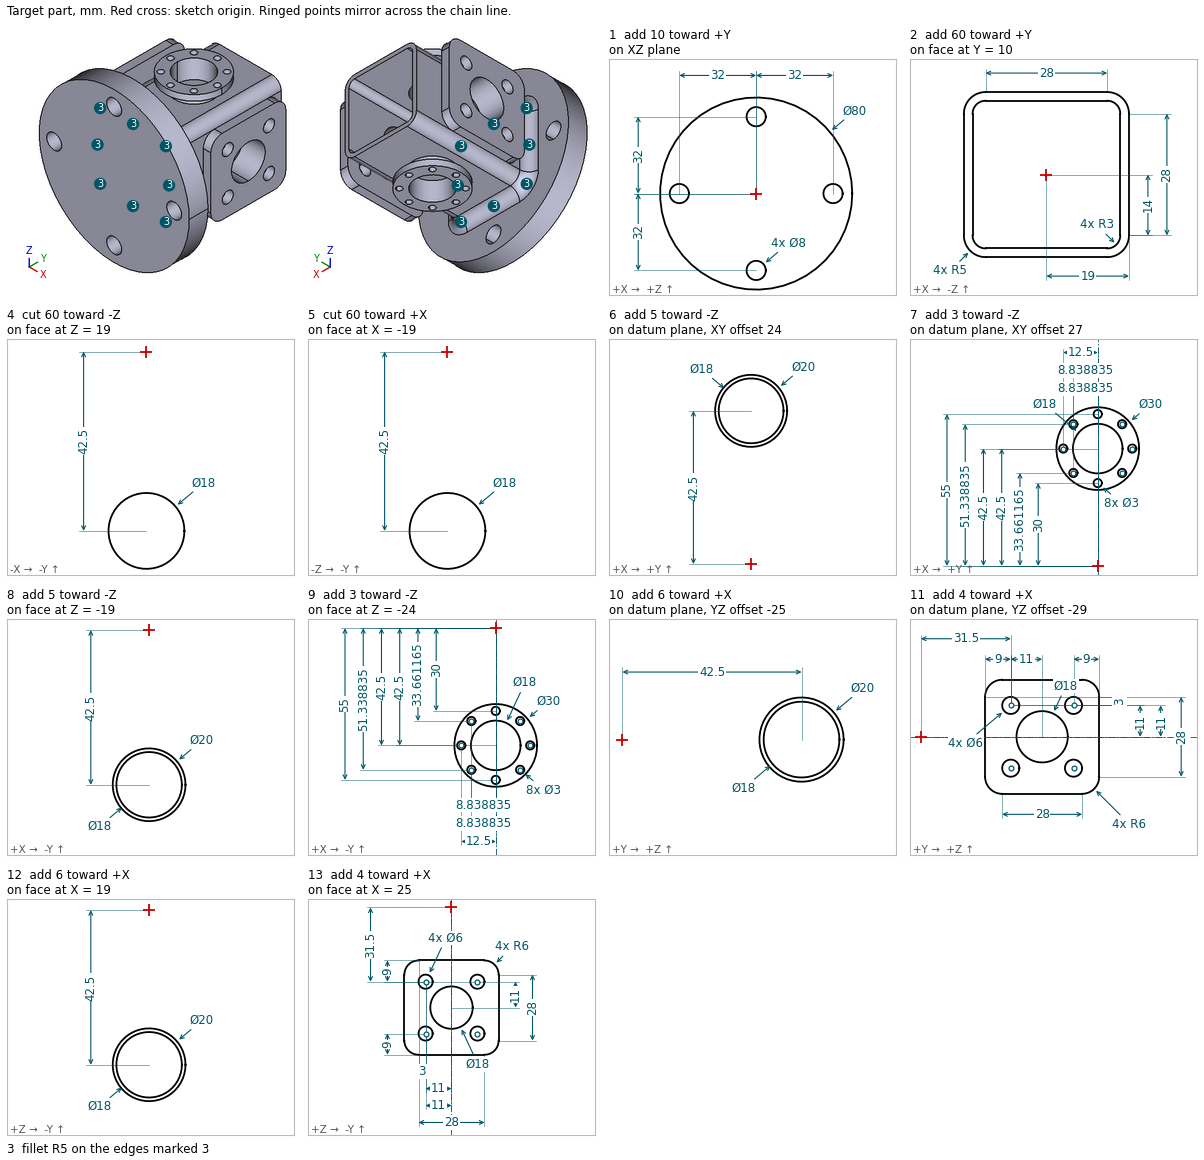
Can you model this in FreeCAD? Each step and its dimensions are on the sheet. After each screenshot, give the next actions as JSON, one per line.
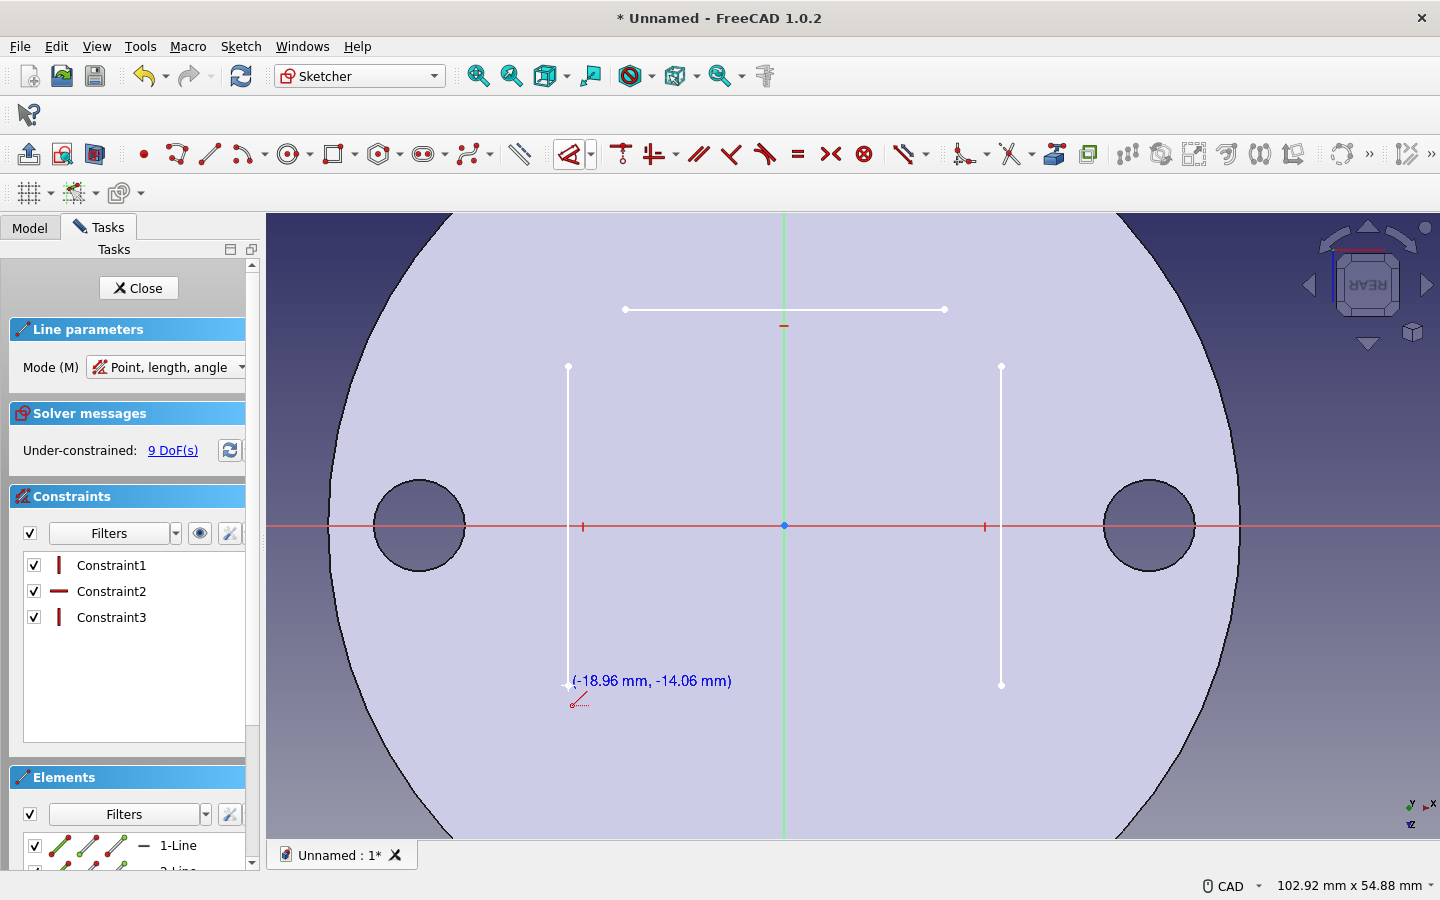
{"action": "left_click", "coordinate": [625, 742]}
{"action": "left_click", "coordinate": [944, 742]}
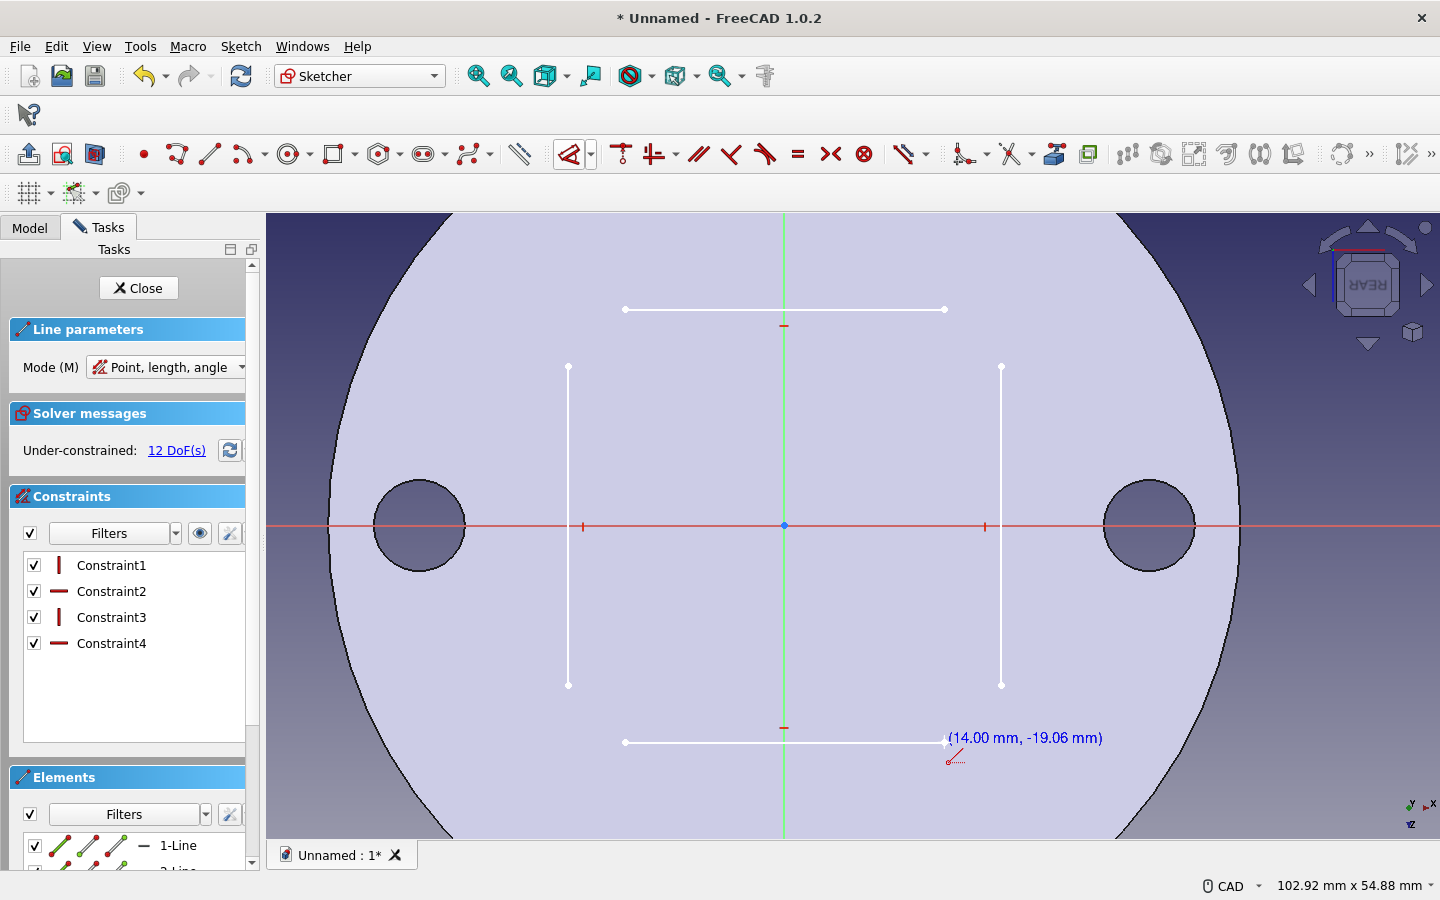
{"action": "key", "text": "g 3 a"}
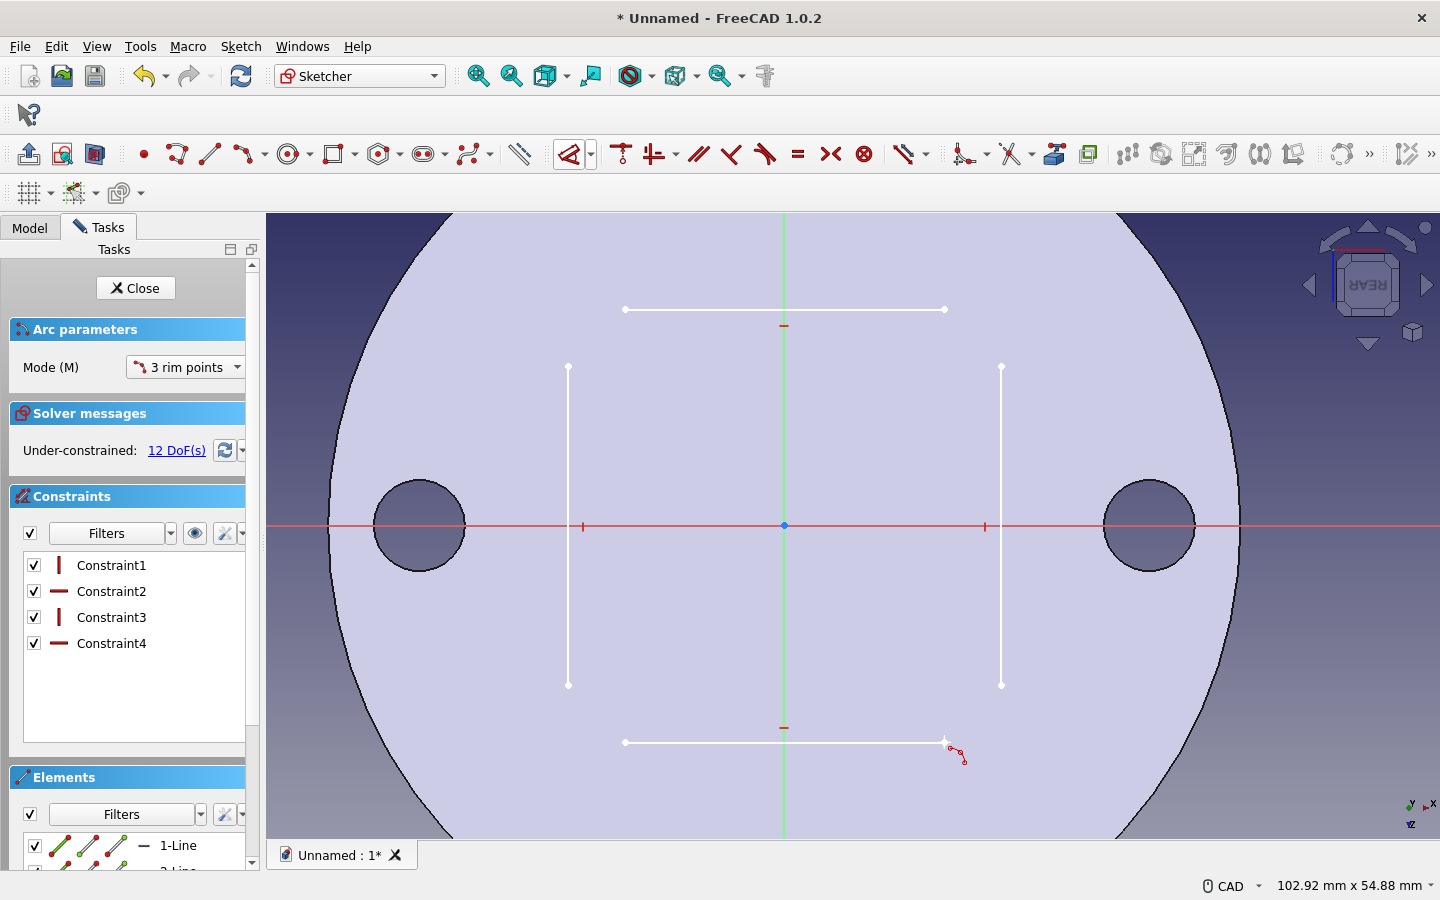
{"action": "left_click", "coordinate": [1001, 367]}
{"action": "left_click", "coordinate": [944, 310]}
{"action": "left_click", "coordinate": [984, 326]}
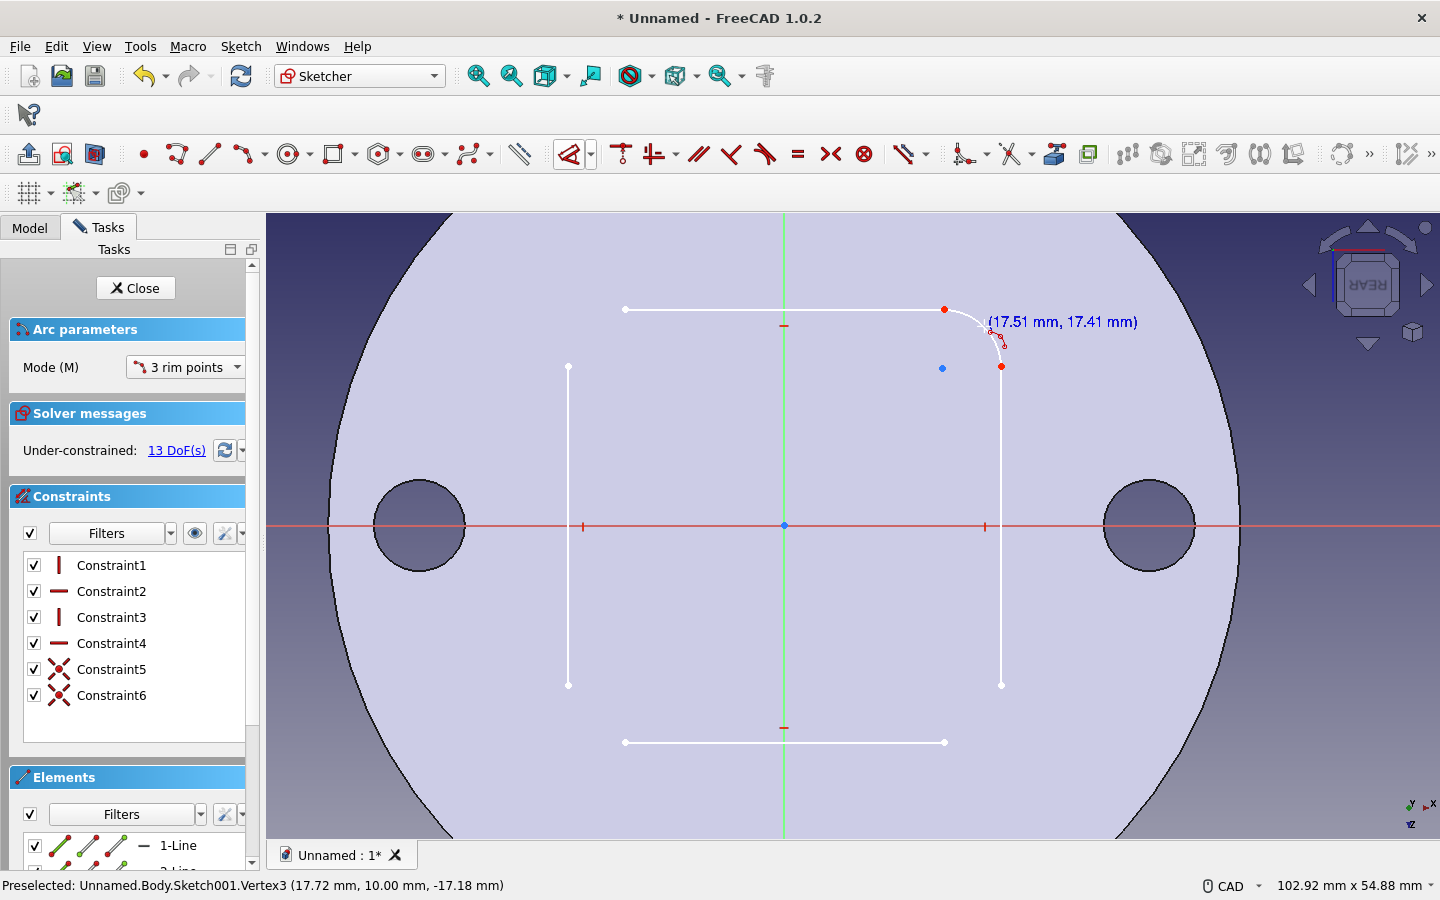
{"action": "left_click", "coordinate": [625, 310]}
{"action": "left_click", "coordinate": [568, 367]}
{"action": "left_click", "coordinate": [584, 326]}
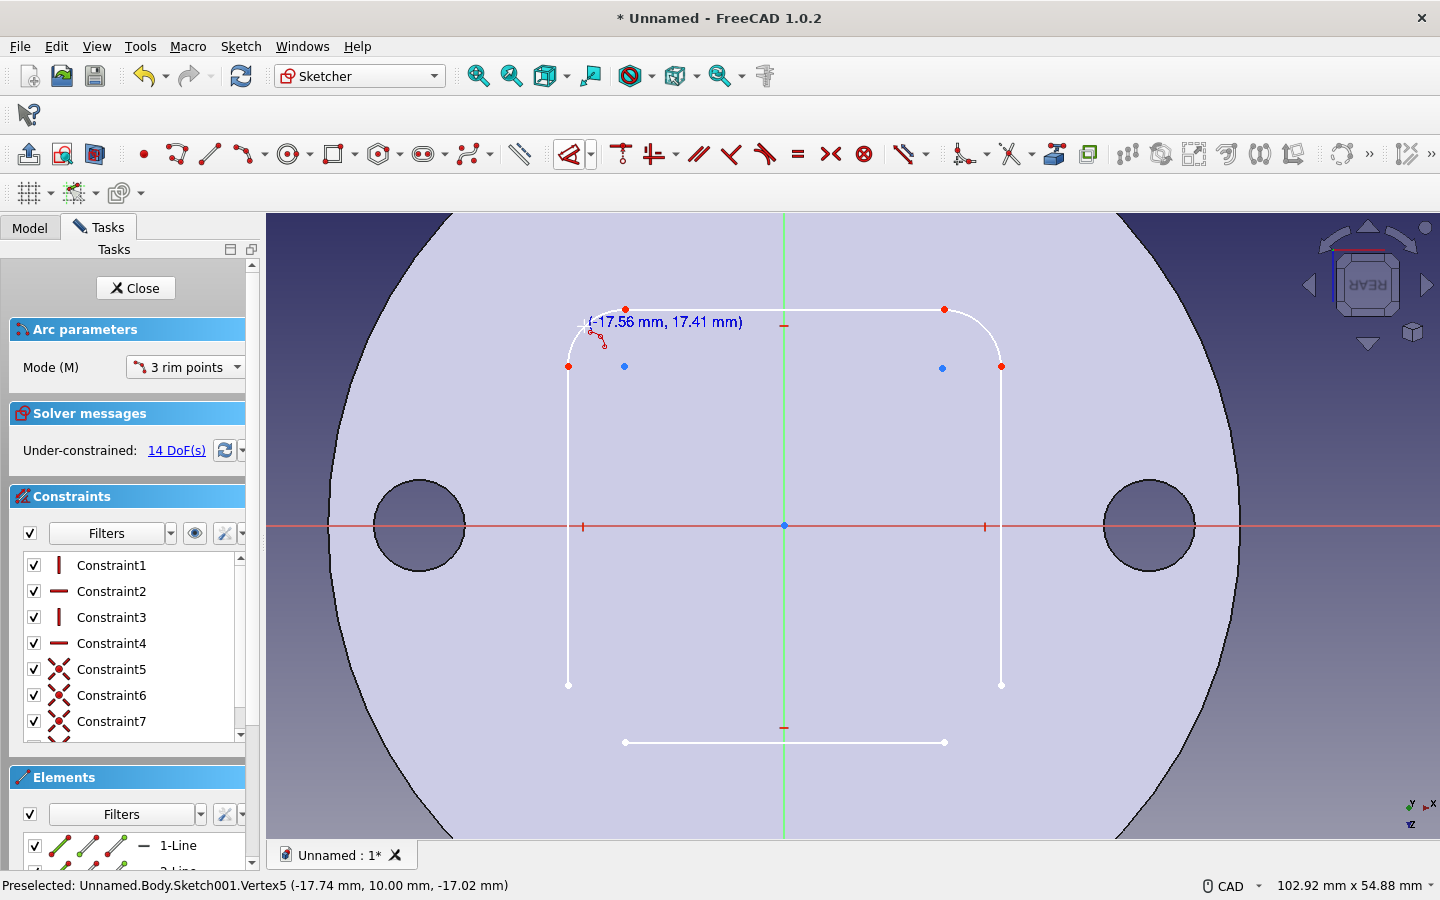
{"action": "left_click", "coordinate": [568, 686]}
{"action": "left_click", "coordinate": [625, 743]}
{"action": "left_click", "coordinate": [584, 726]}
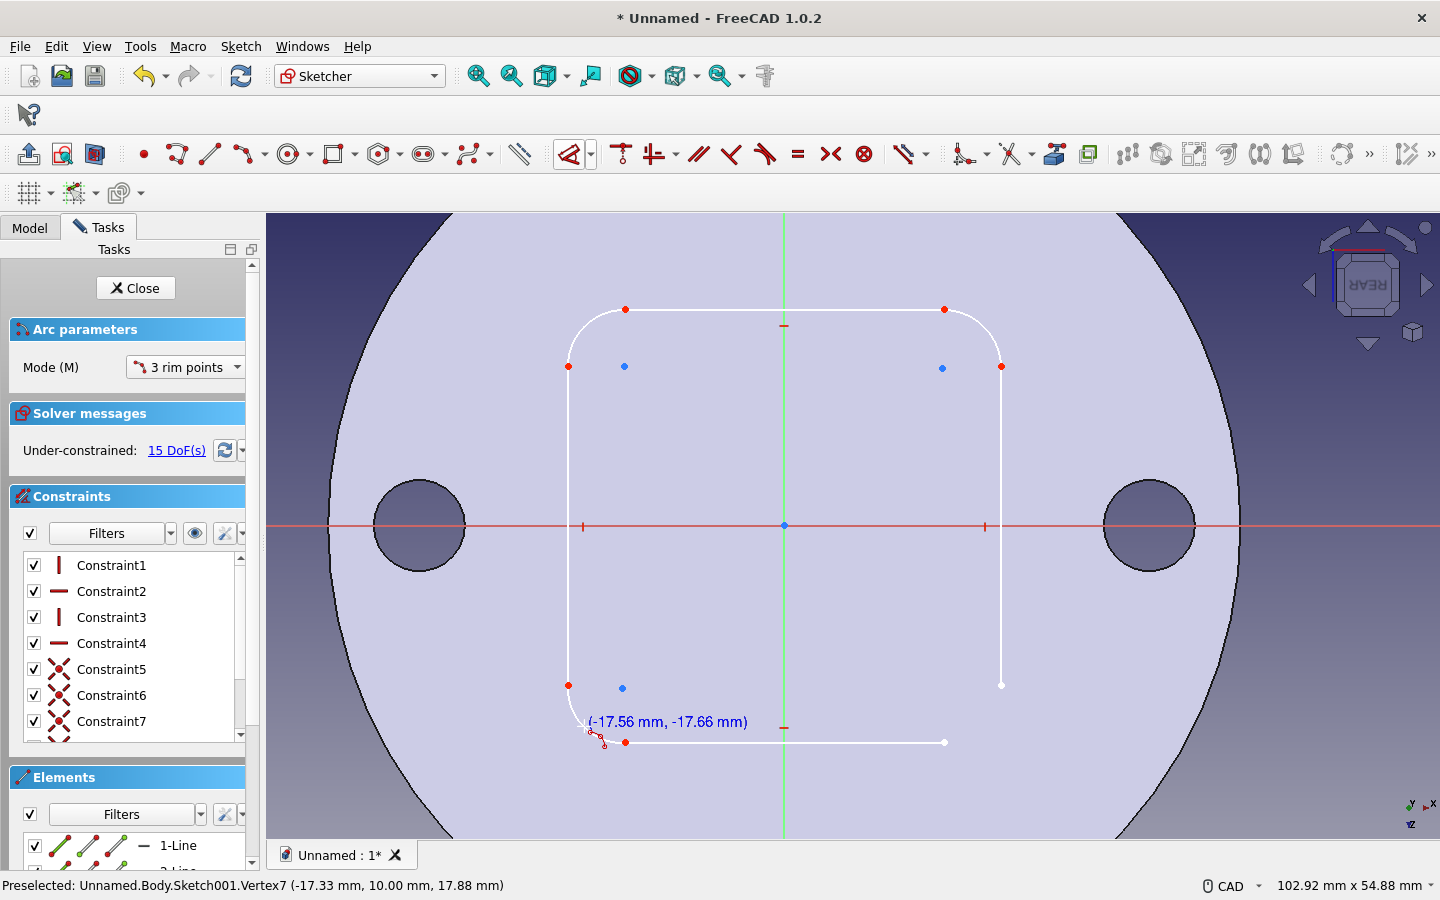
{"action": "left_click", "coordinate": [944, 743]}
{"action": "left_click", "coordinate": [1001, 686]}
{"action": "left_click", "coordinate": [984, 726]}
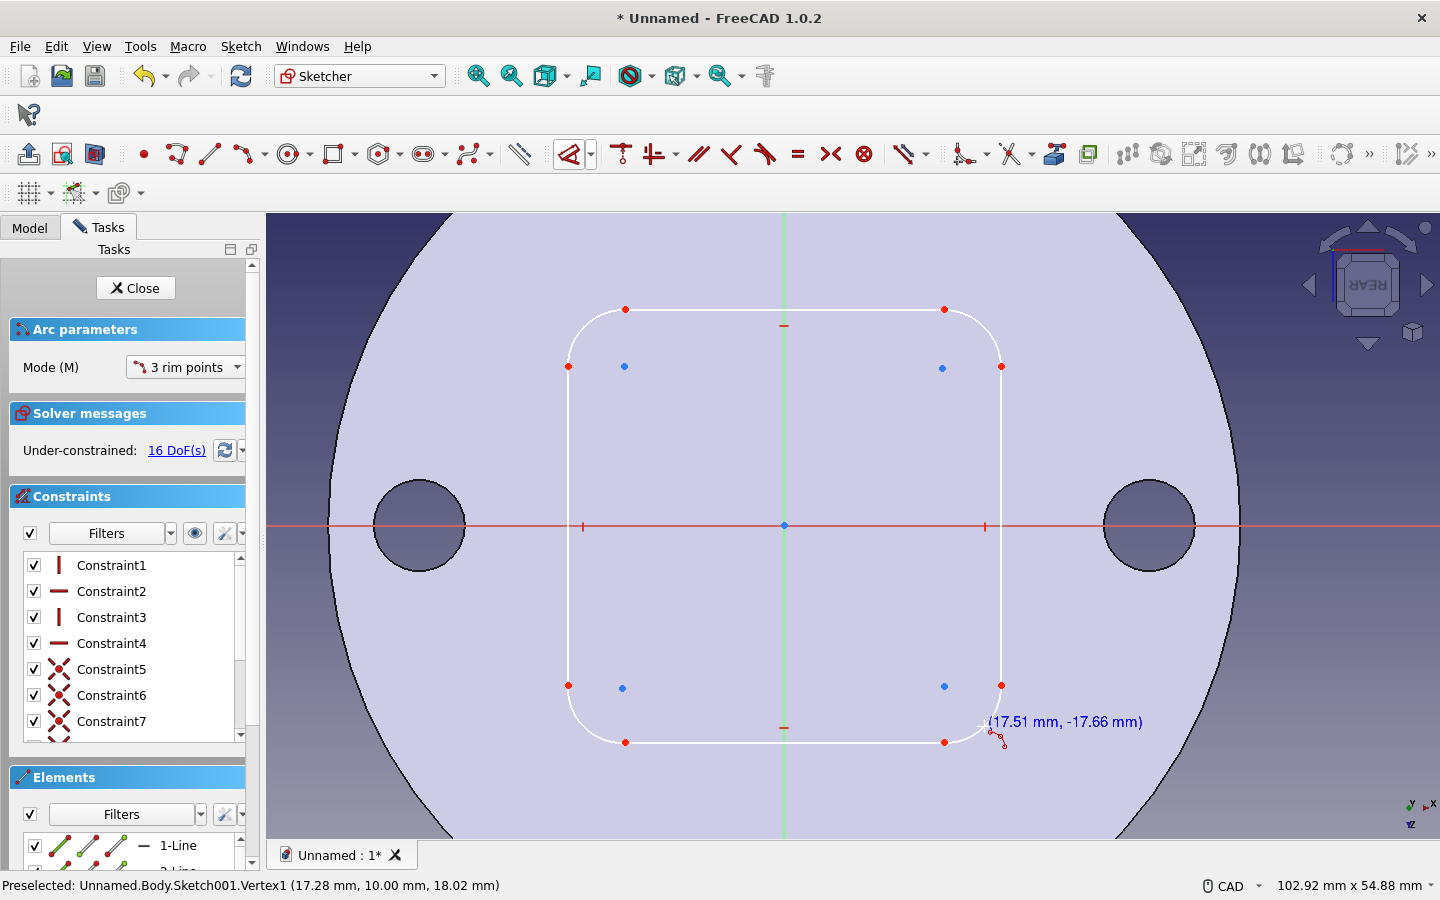
{"action": "key", "text": "g l"}